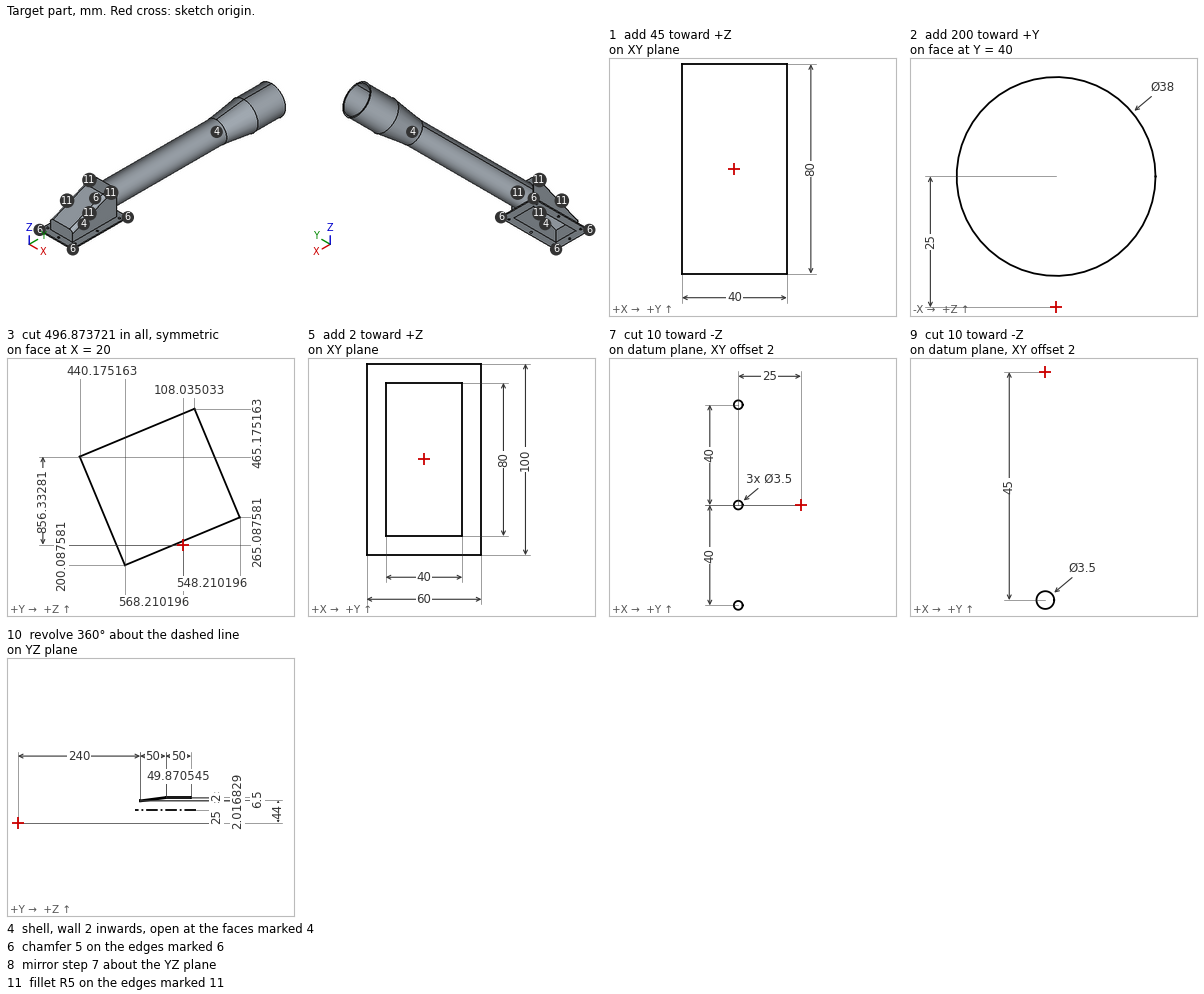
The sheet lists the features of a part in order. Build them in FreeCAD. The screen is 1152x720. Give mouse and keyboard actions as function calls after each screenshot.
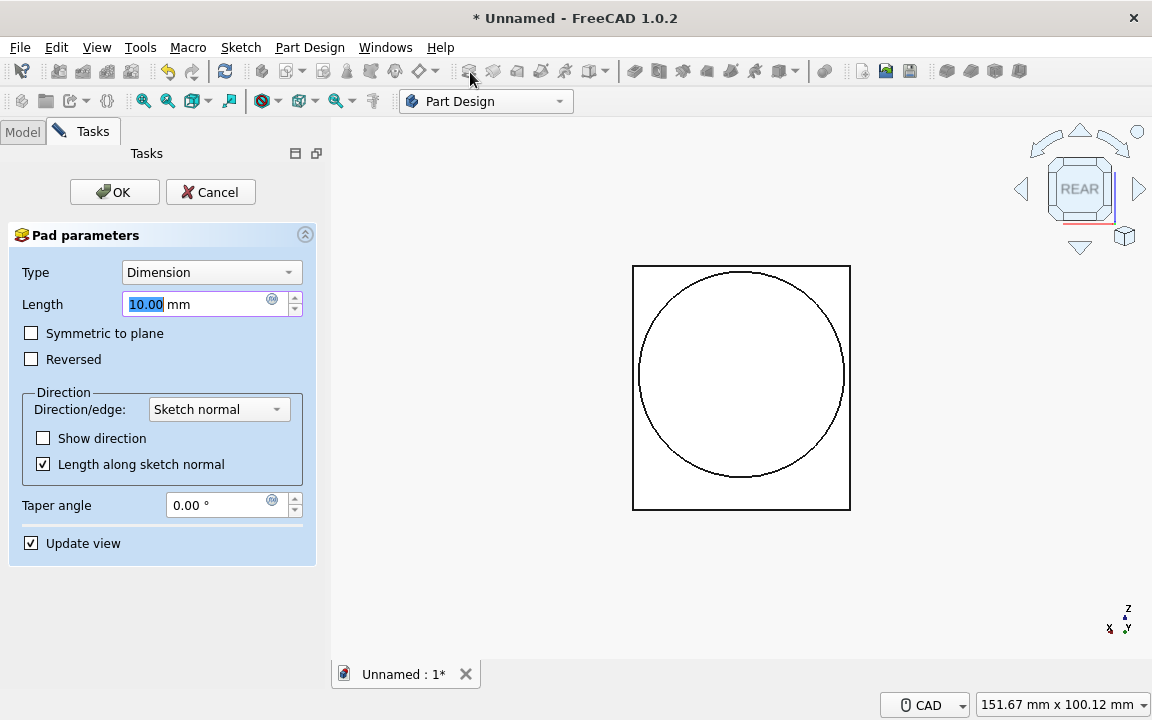
text(200)
key(Tab)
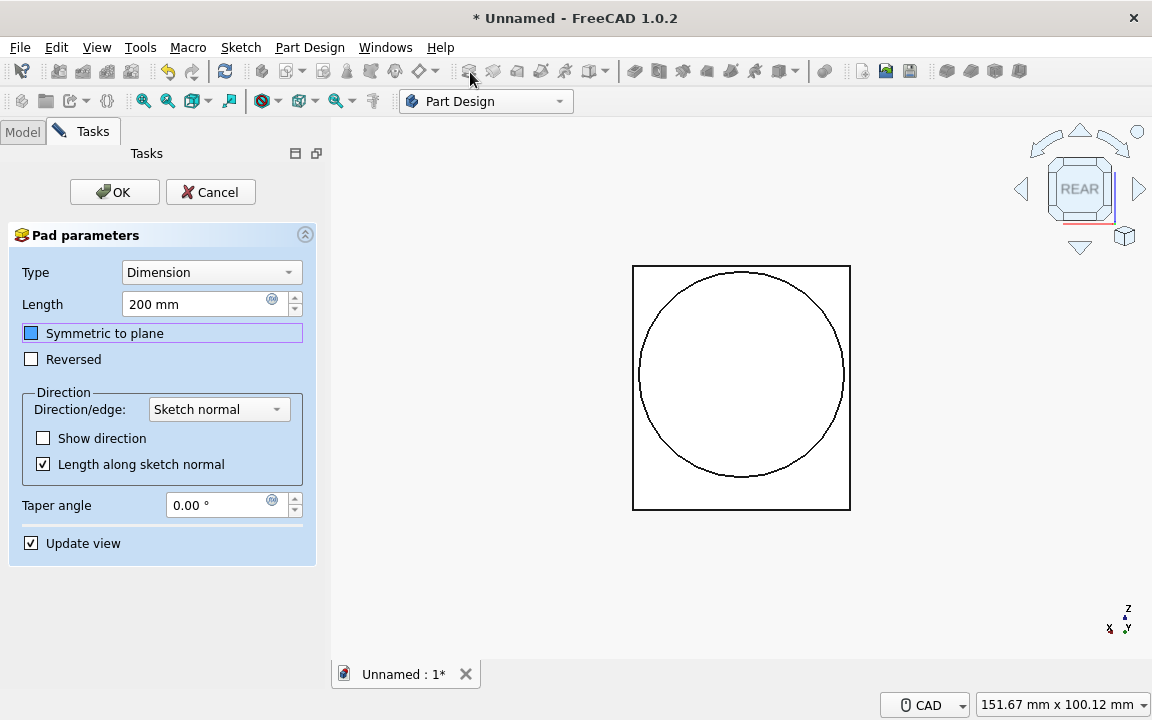
click(115, 192)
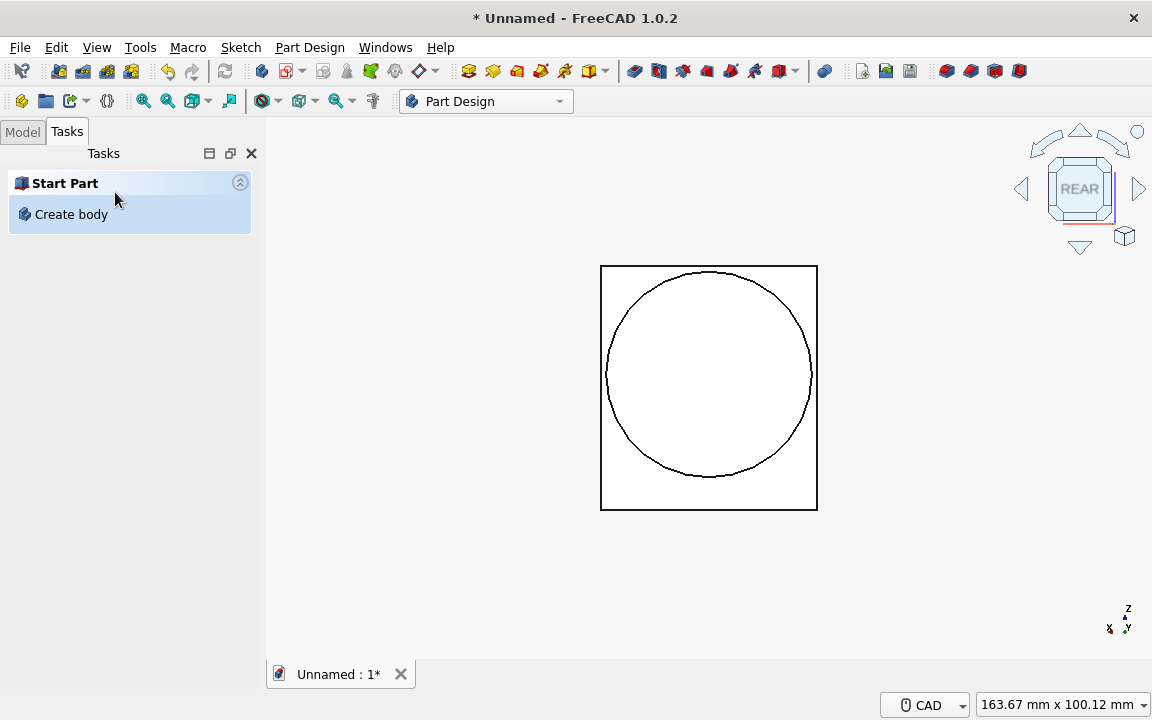
key(0)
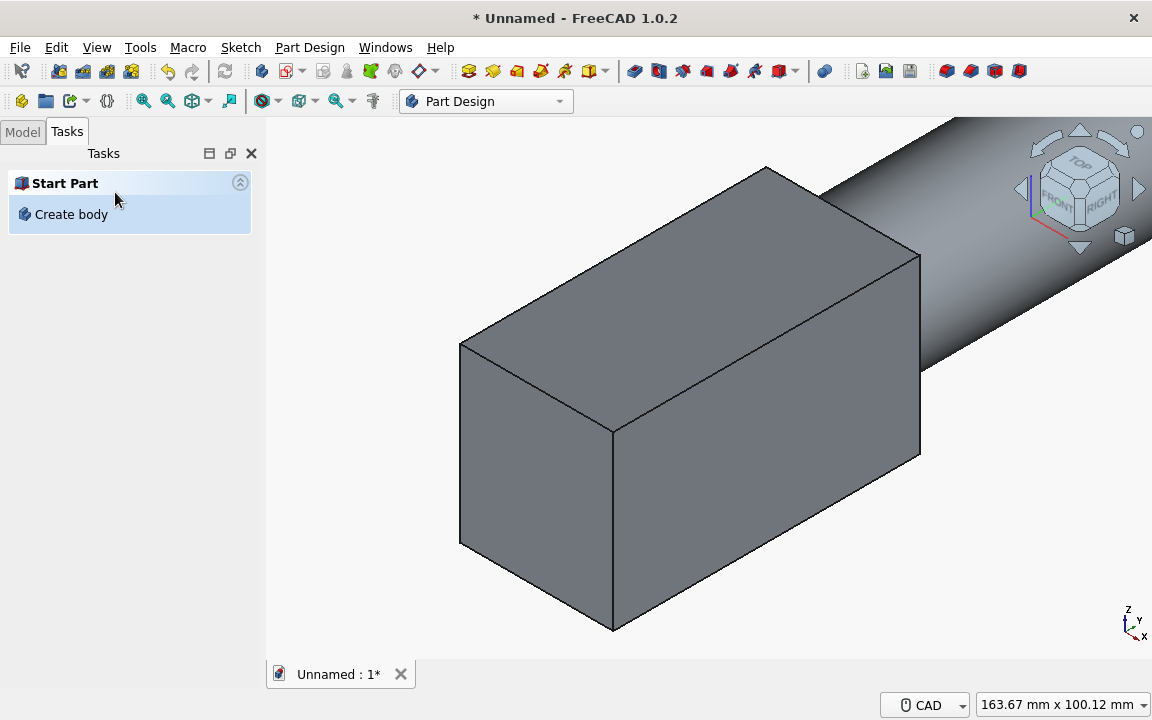
key(v)
key(f)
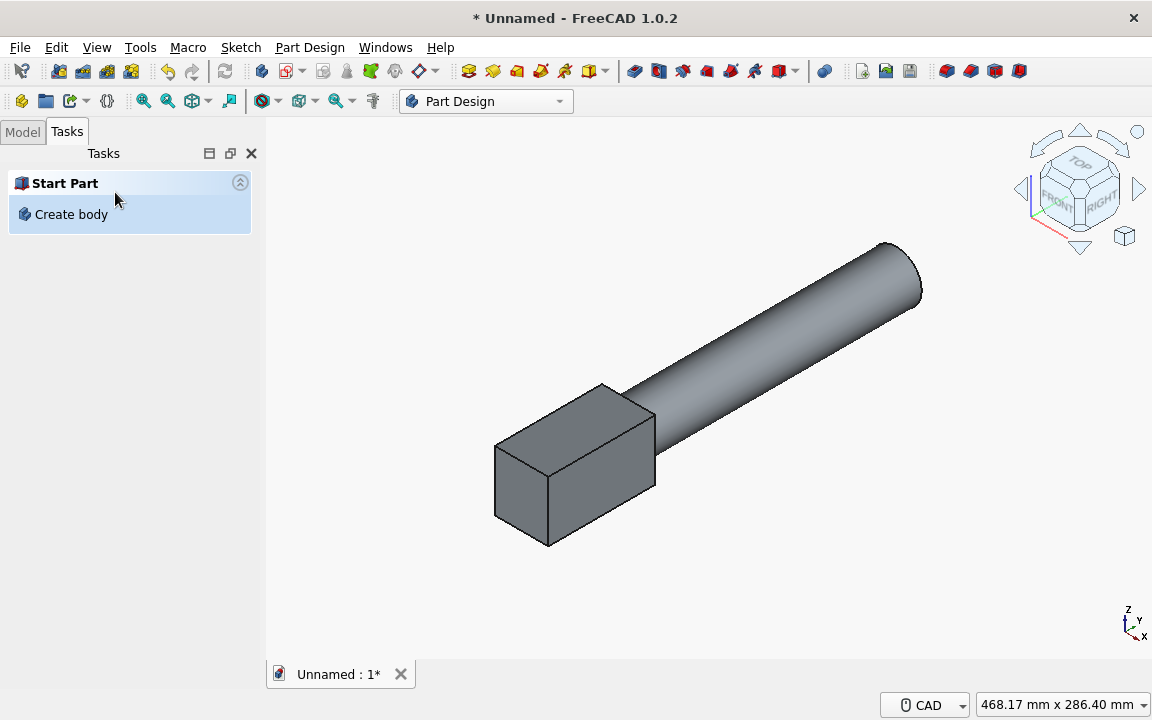
click(617, 471)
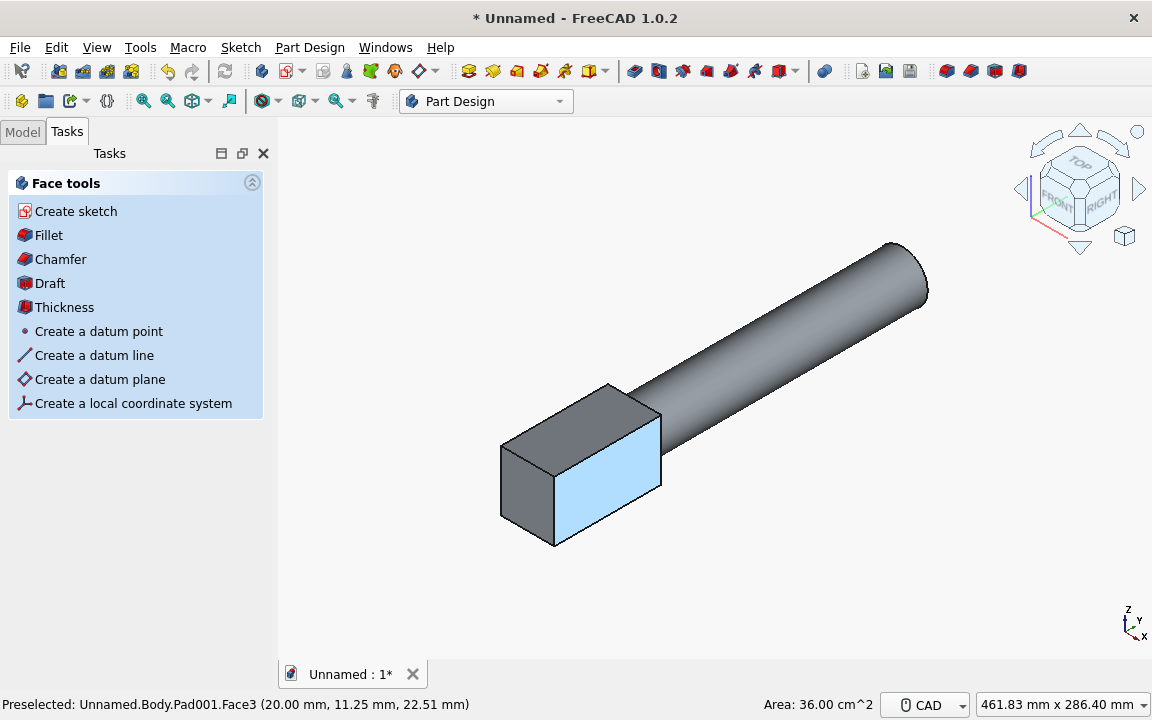
click(286, 72)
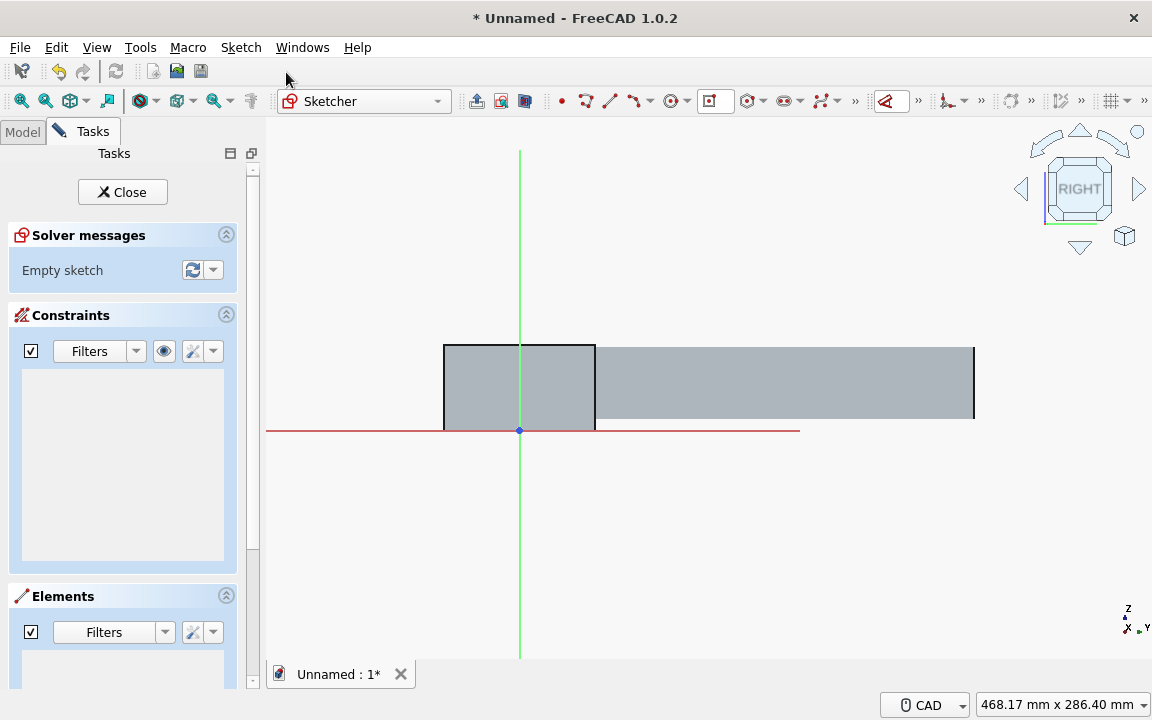
scroll(710, 515, down, 11)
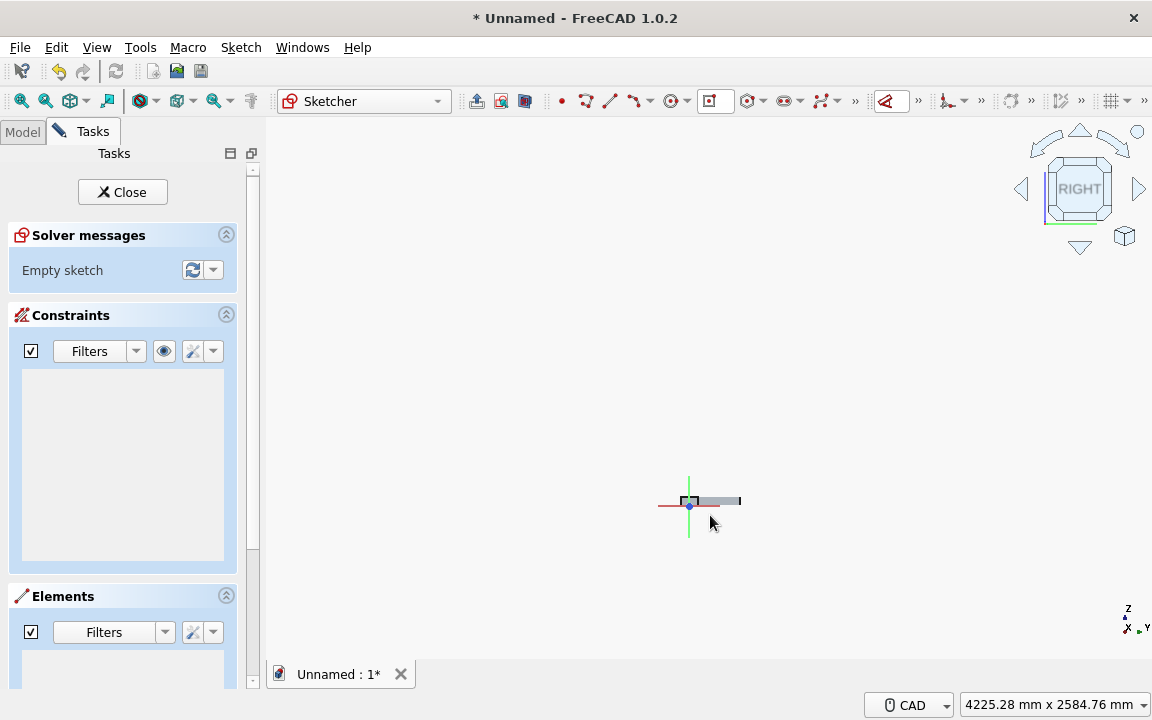
click(586, 102)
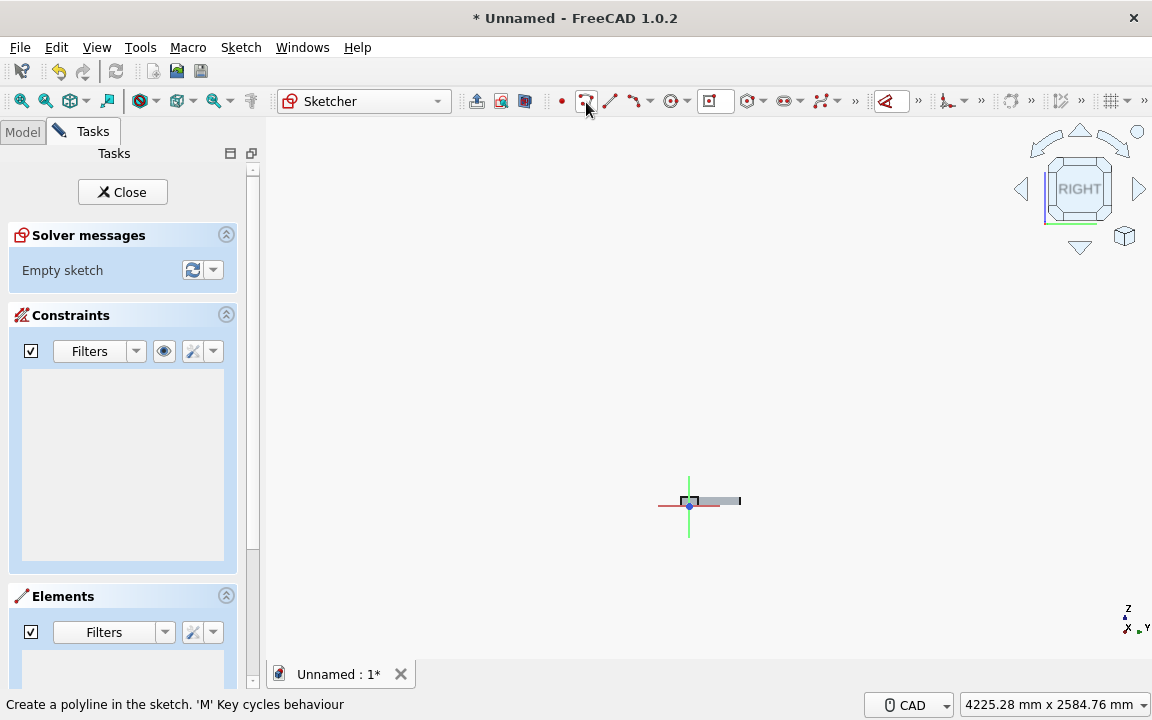
click(570, 548)
click(804, 451)
click(712, 229)
click(478, 327)
click(570, 549)
key(Escape)
key(Escape)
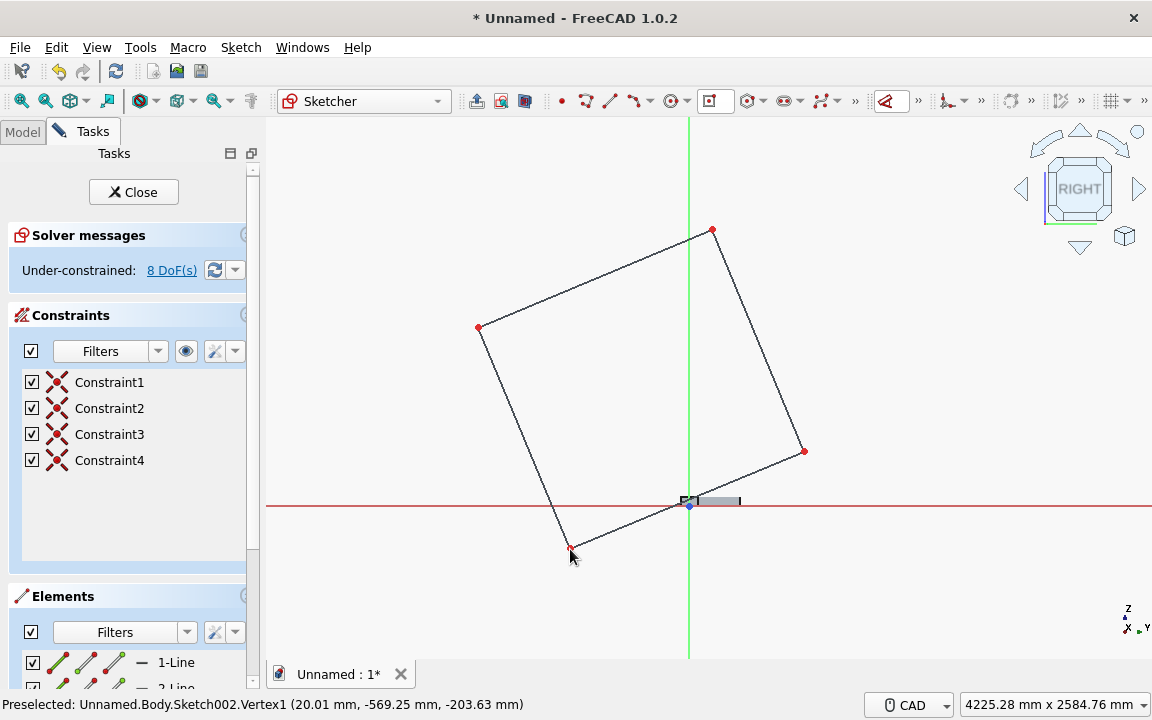
key(d)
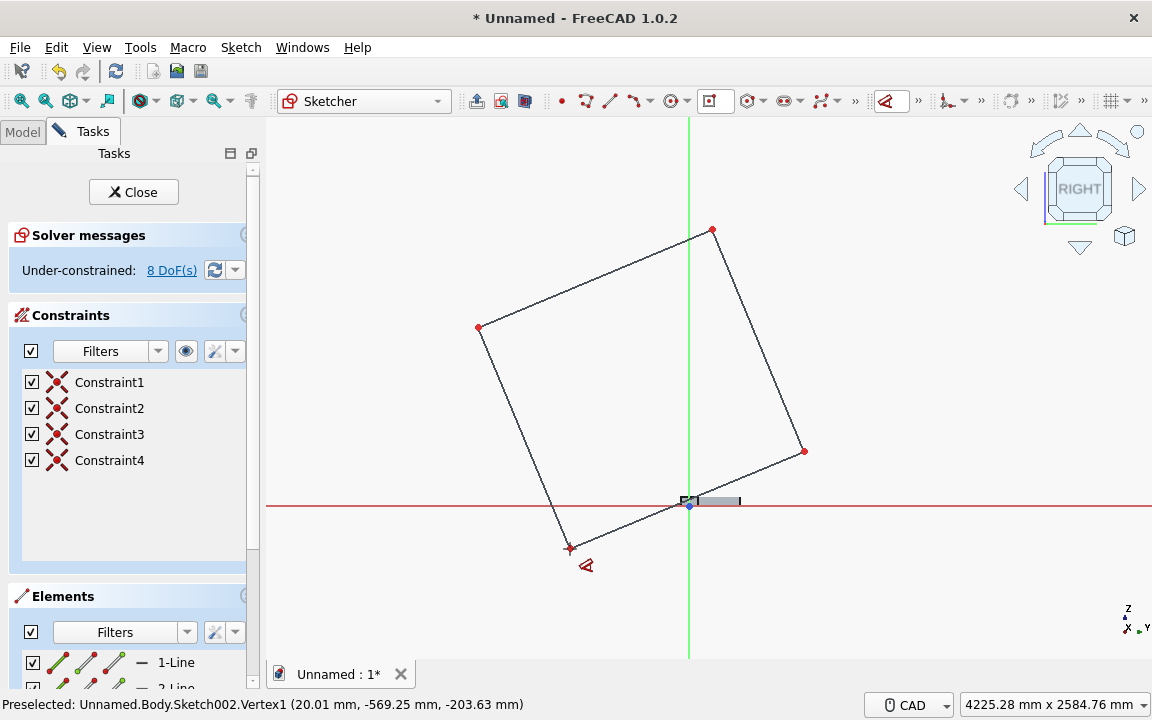
click(478, 328)
click(444, 417)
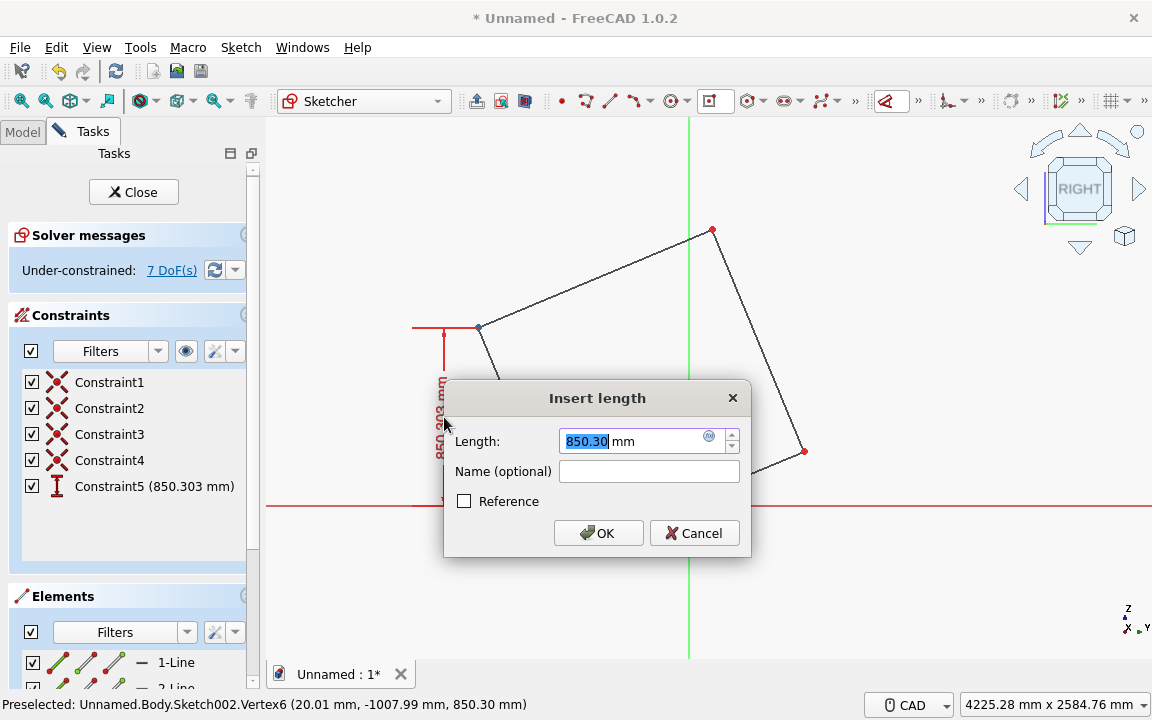
text(856.33281)
key(Return)